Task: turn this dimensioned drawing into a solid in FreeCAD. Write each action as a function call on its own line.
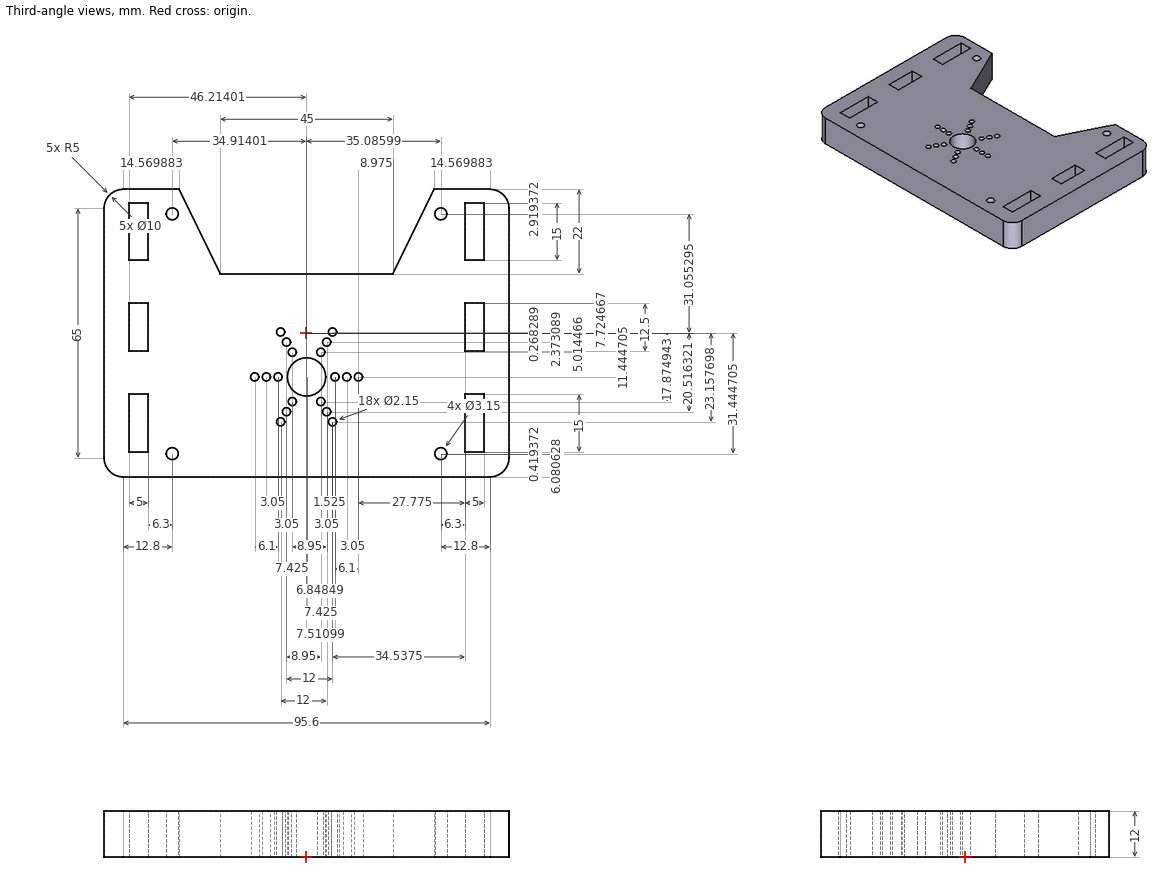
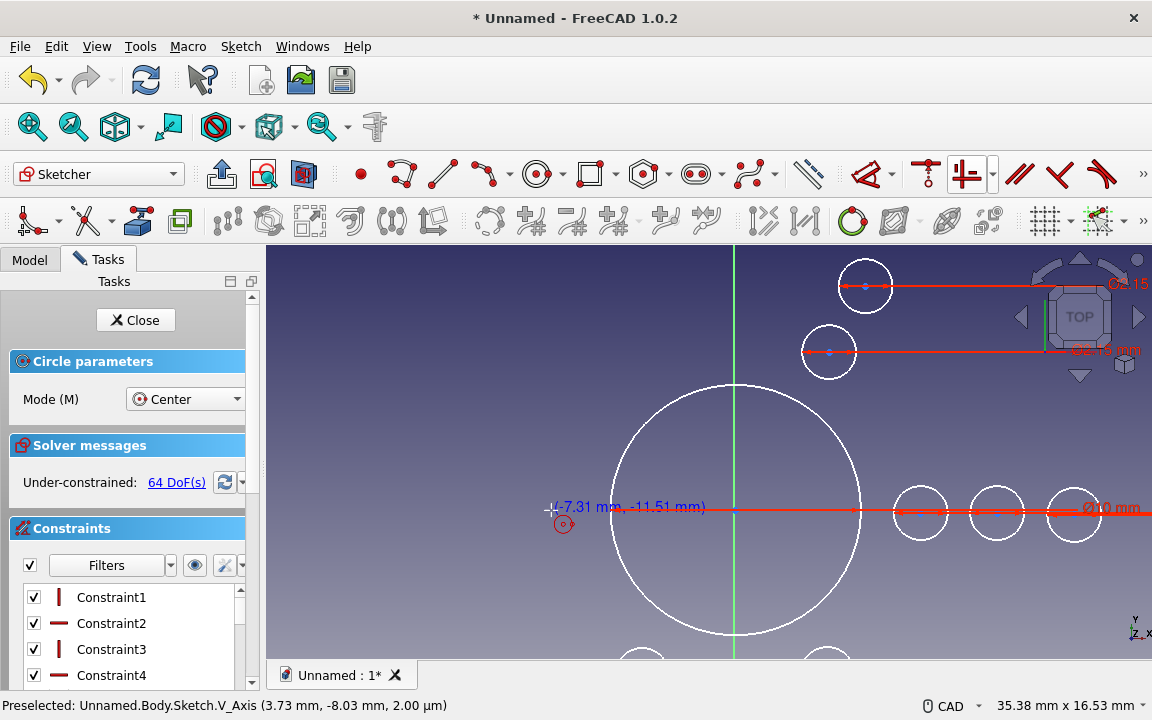
scroll(626, 488, down, 10)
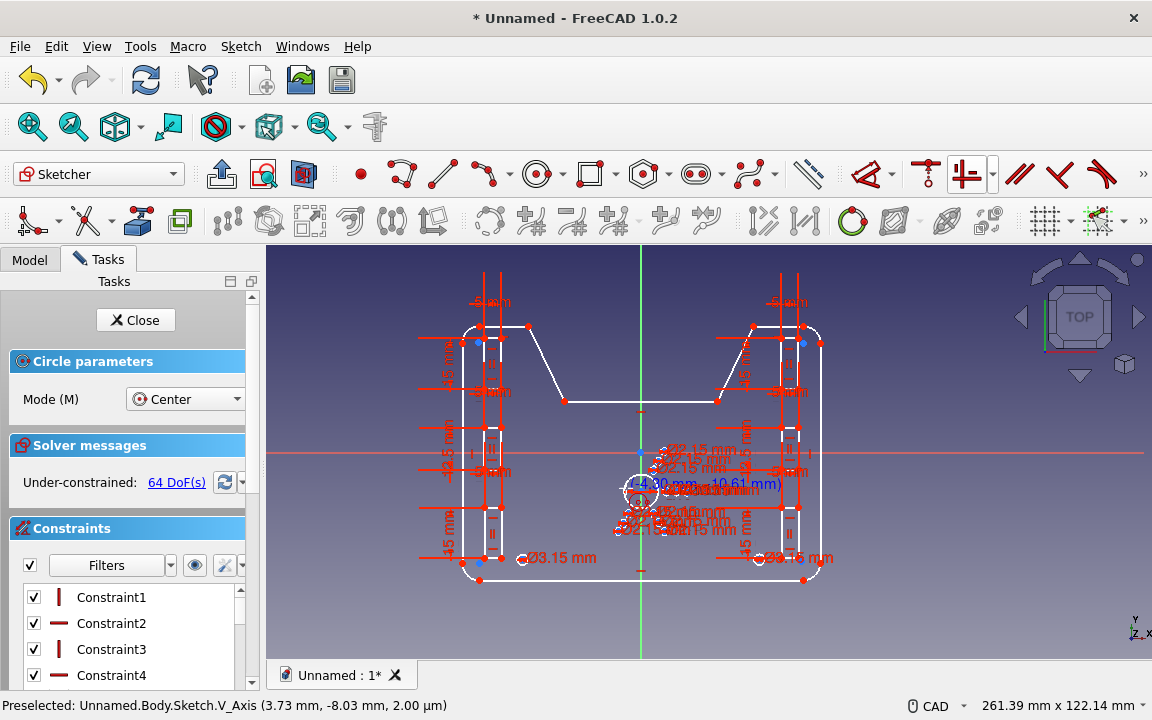
scroll(616, 491, up, 4)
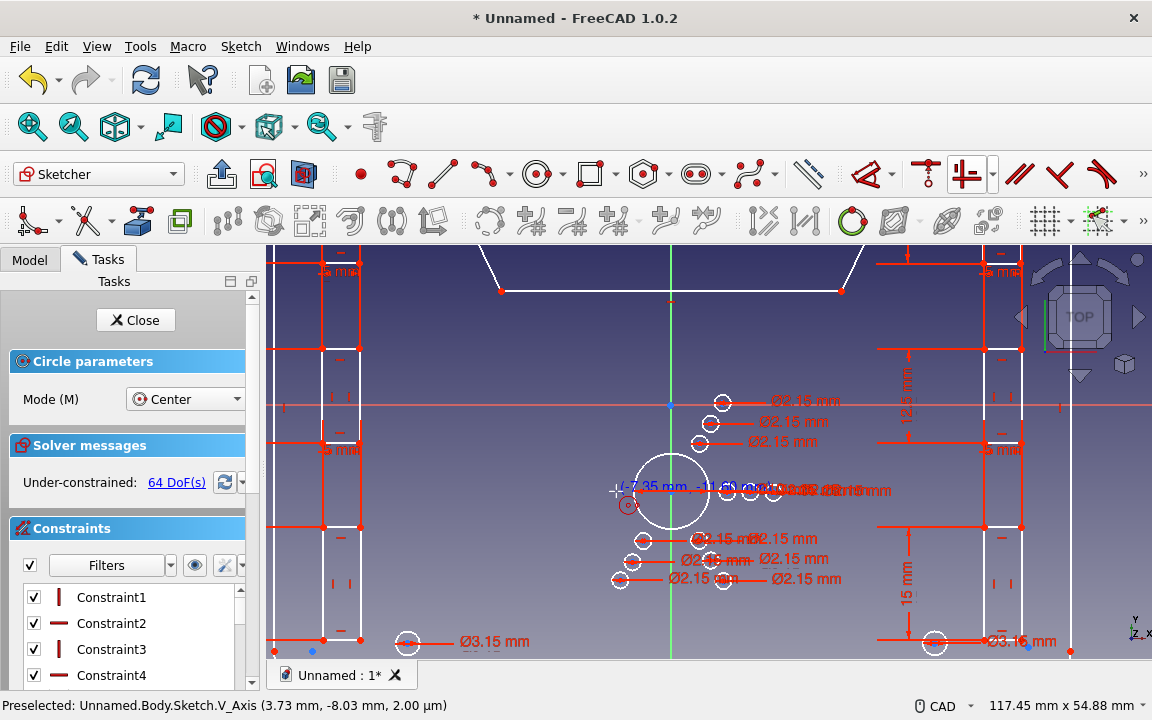
click(616, 491)
move(610, 486)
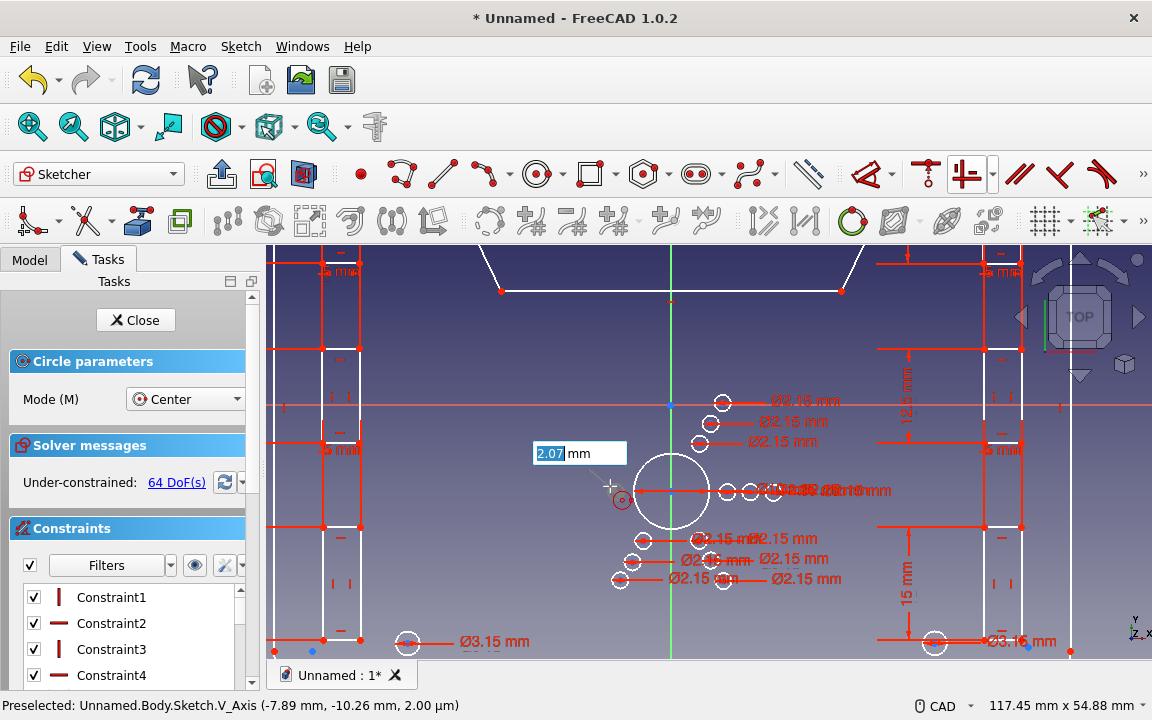
text(2.15)
key(Return)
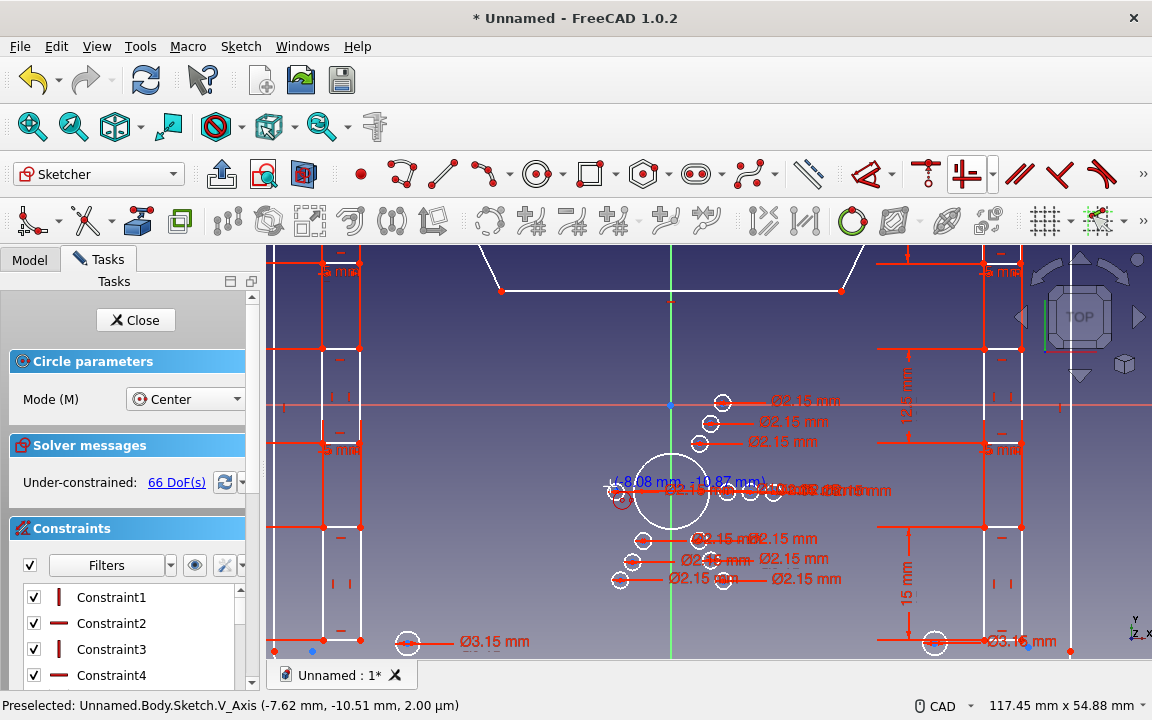
scroll(593, 491, up, 6)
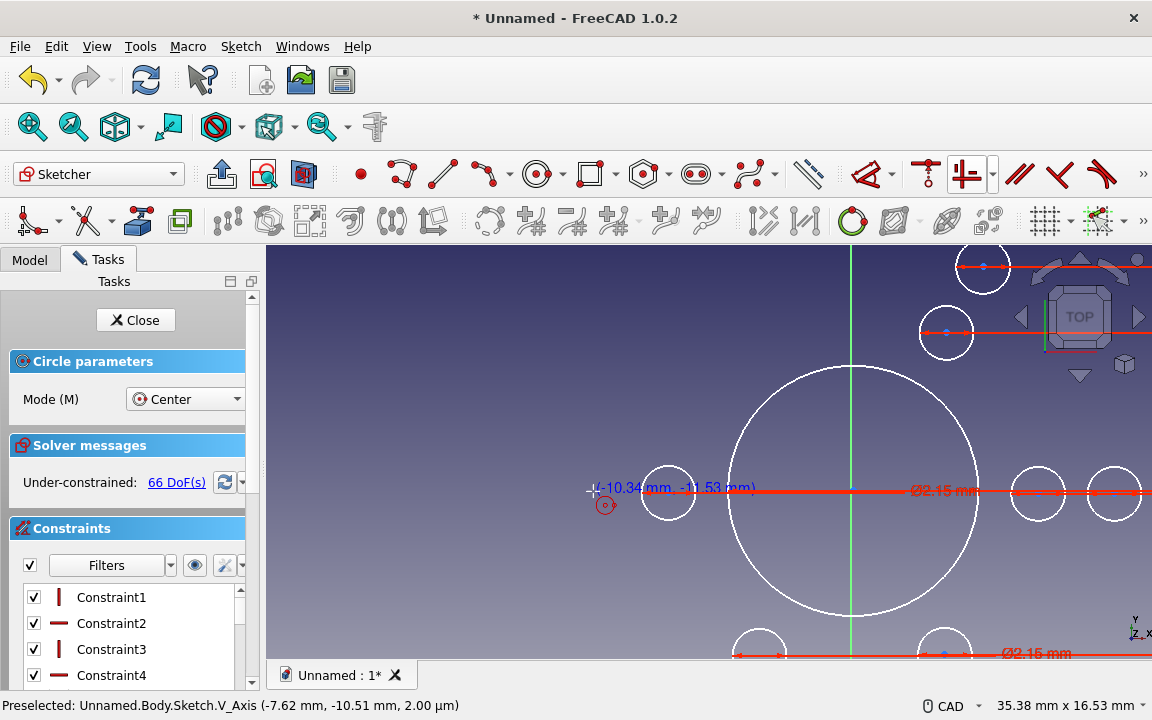
scroll(607, 491, down, 10)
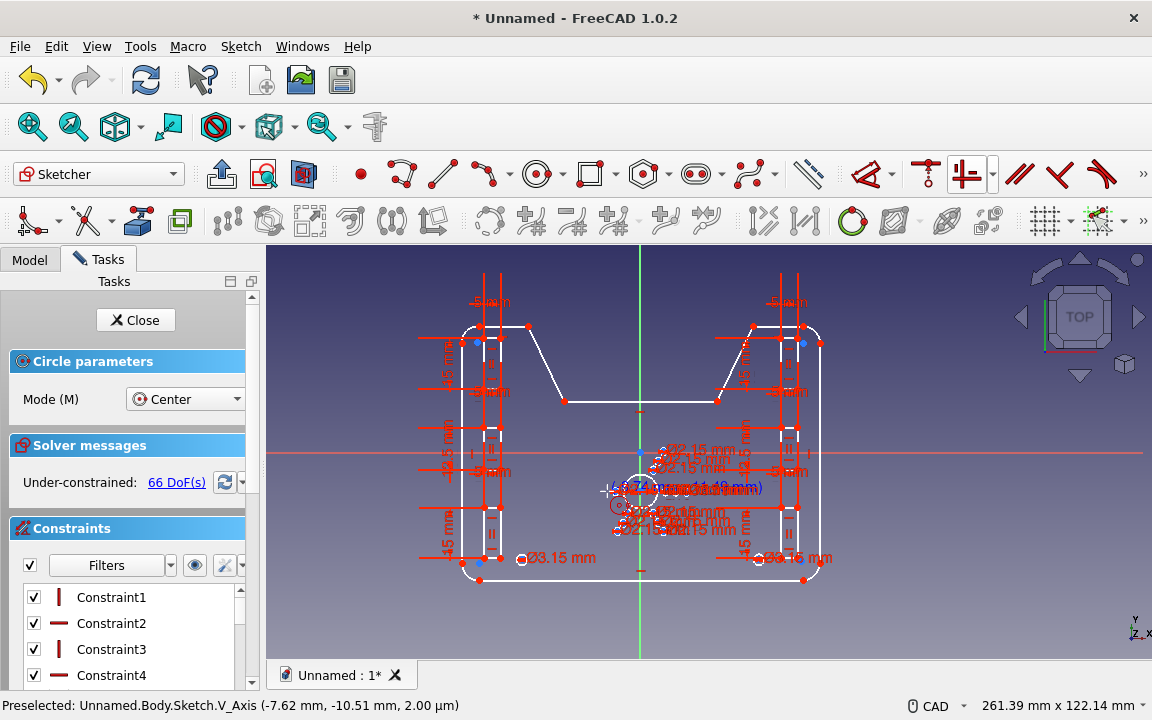
scroll(605, 491, up, 5)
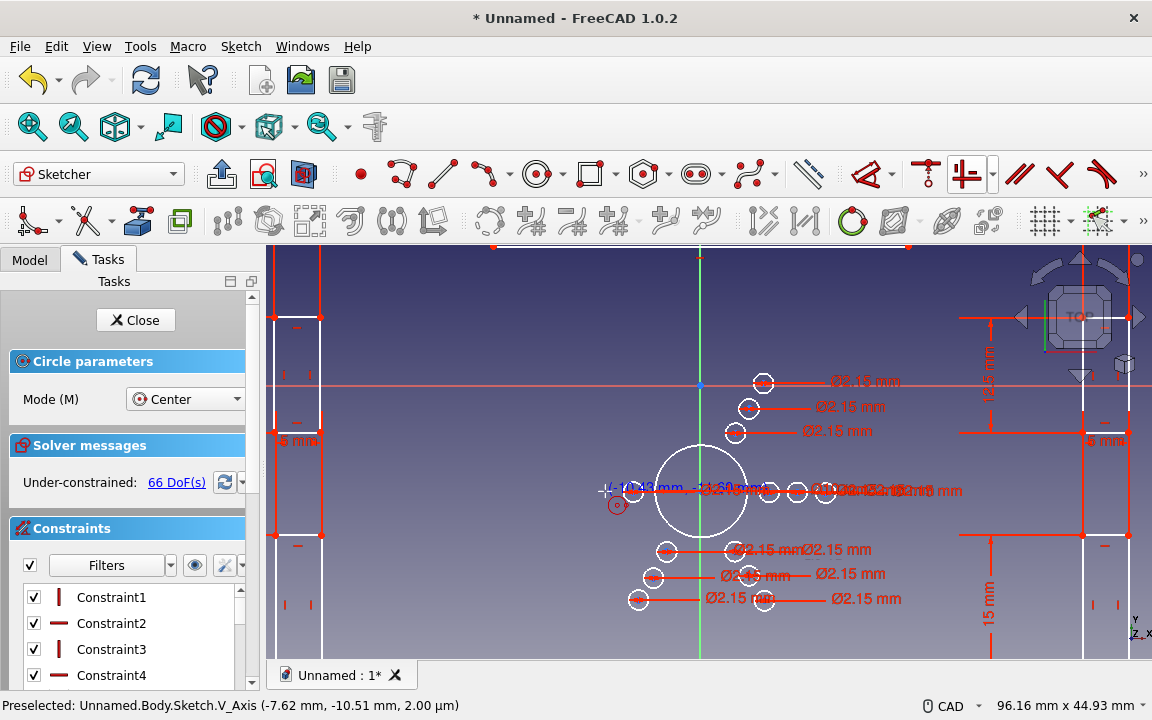
click(605, 491)
move(598, 484)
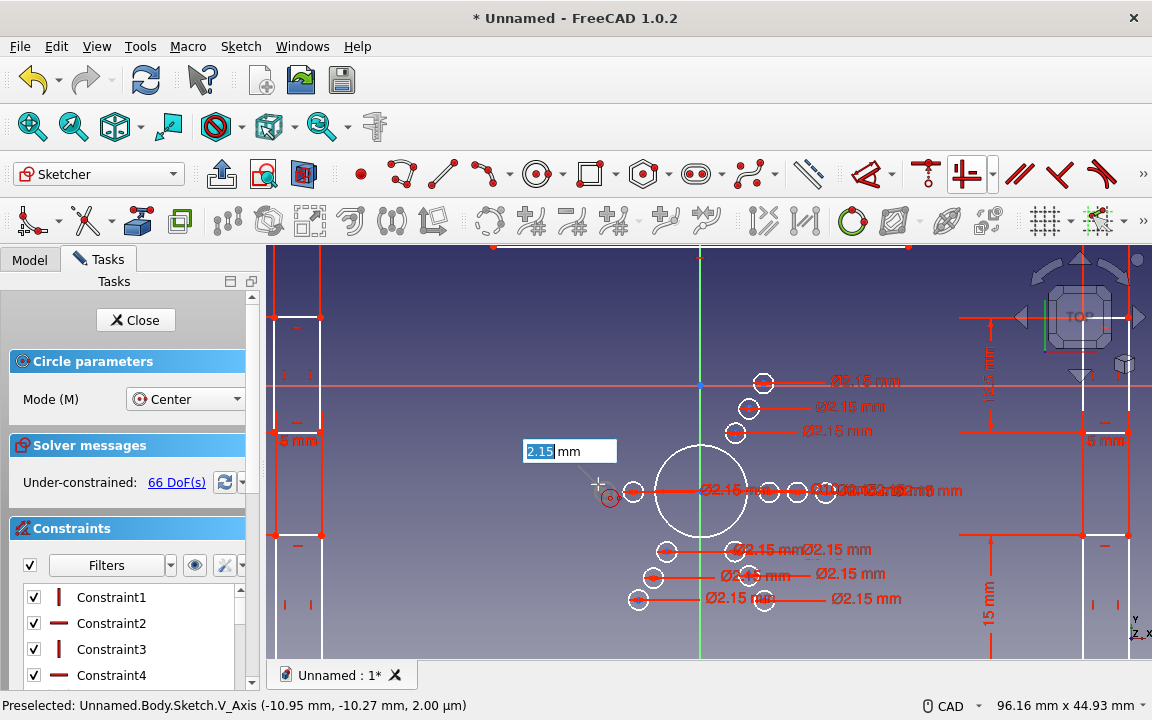
text(2.15)
key(Return)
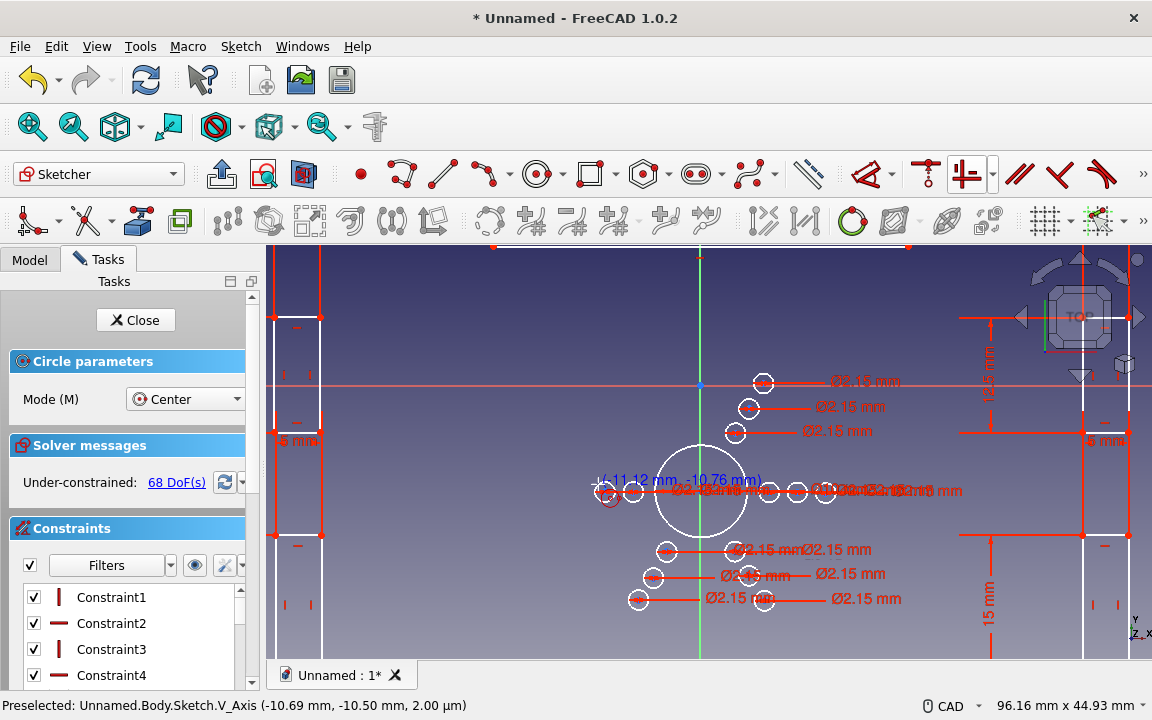
scroll(577, 491, up, 5)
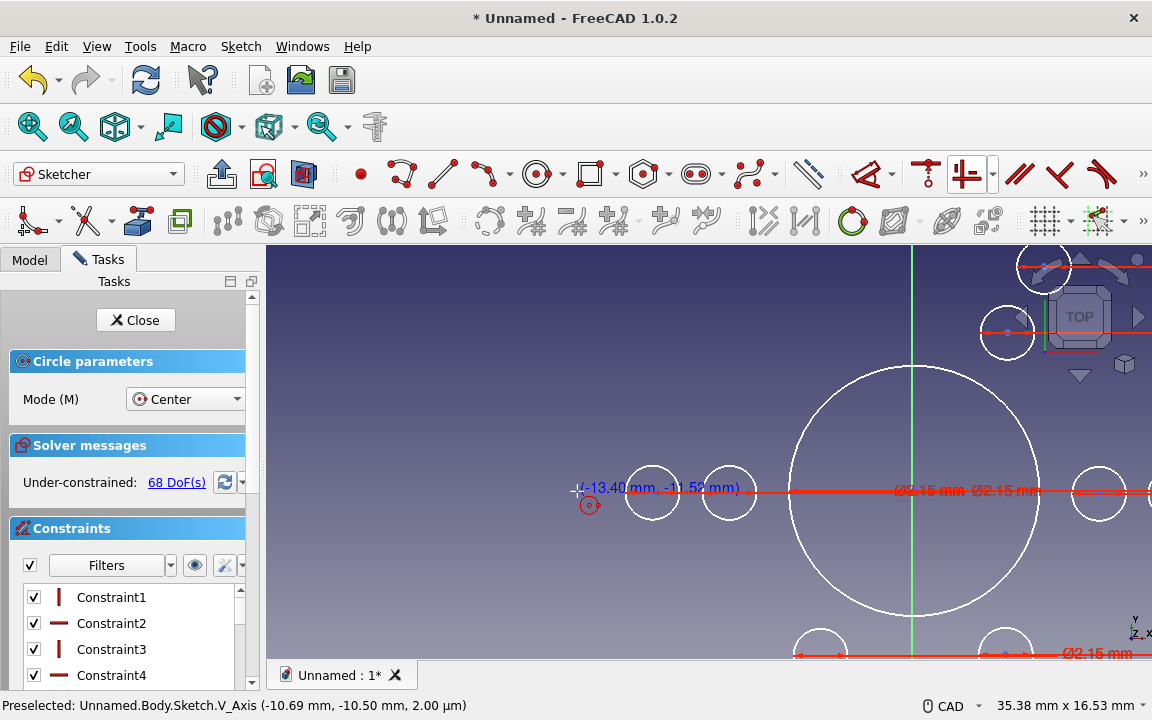
scroll(598, 491, down, 10)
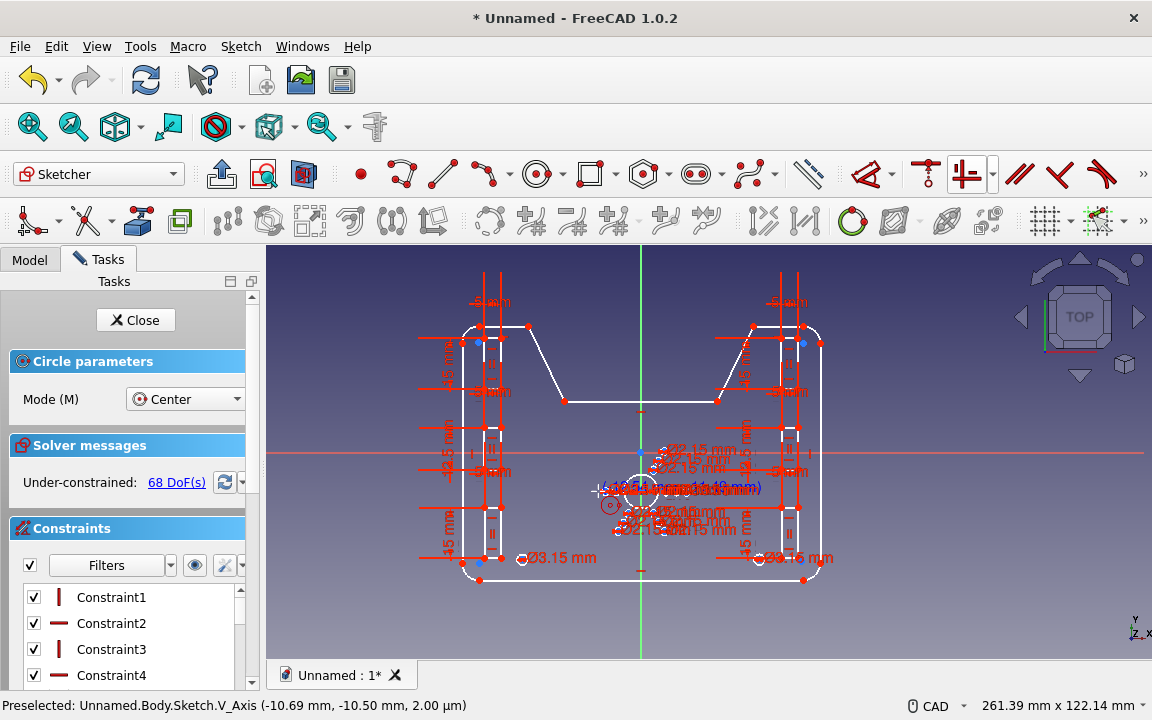
scroll(595, 491, up, 5)